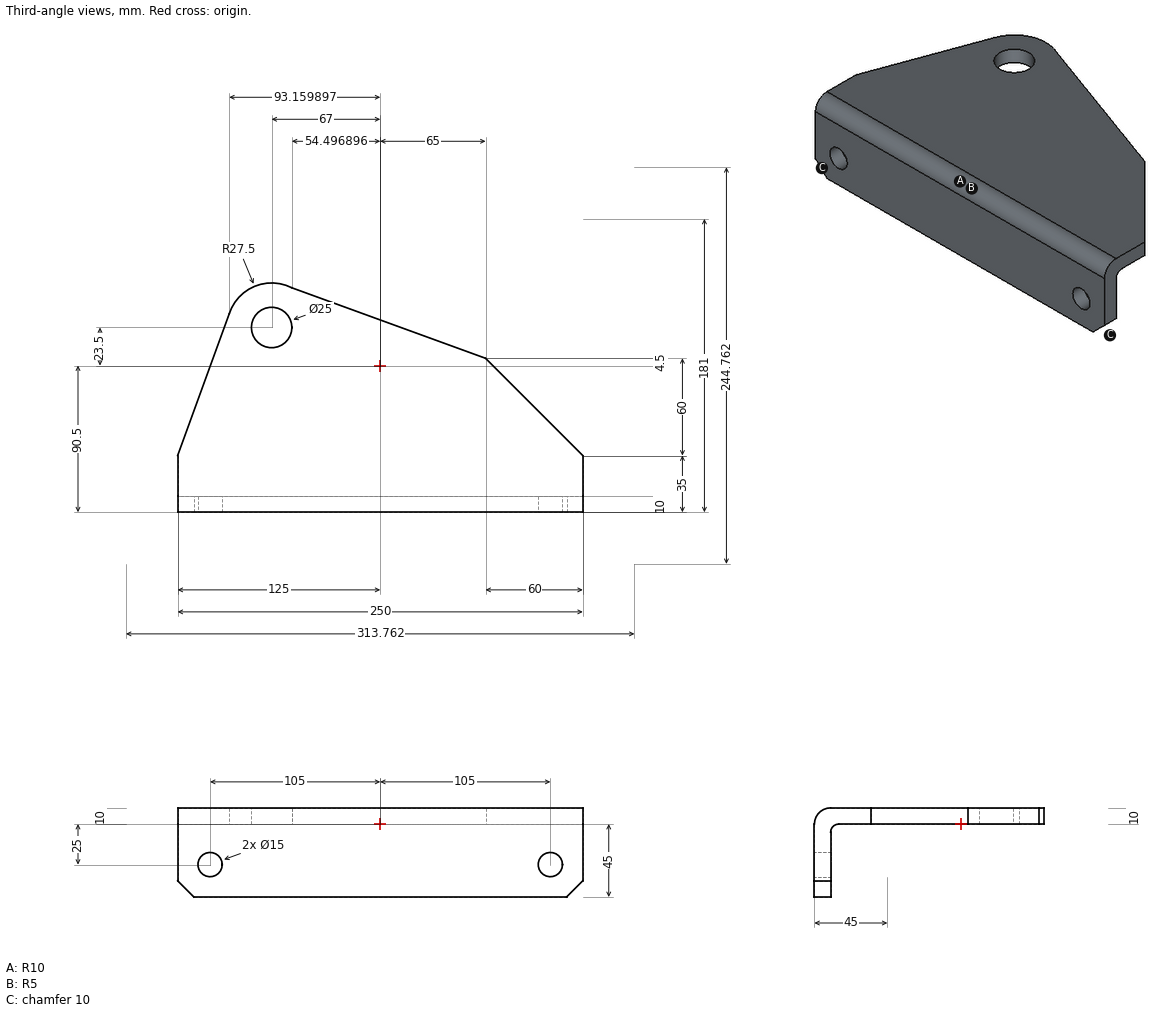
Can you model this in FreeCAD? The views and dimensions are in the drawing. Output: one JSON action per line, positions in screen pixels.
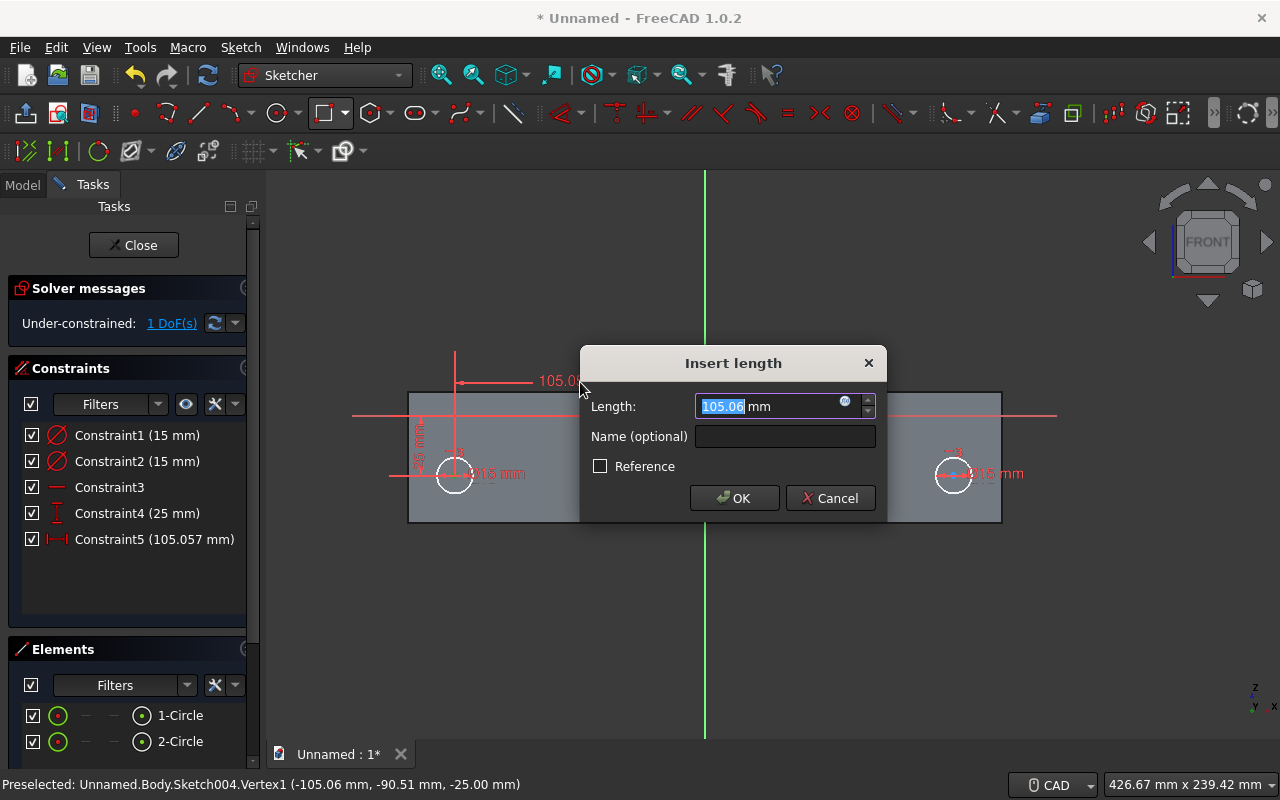
{"action": "type", "text": "105"}
{"action": "key", "text": "Return"}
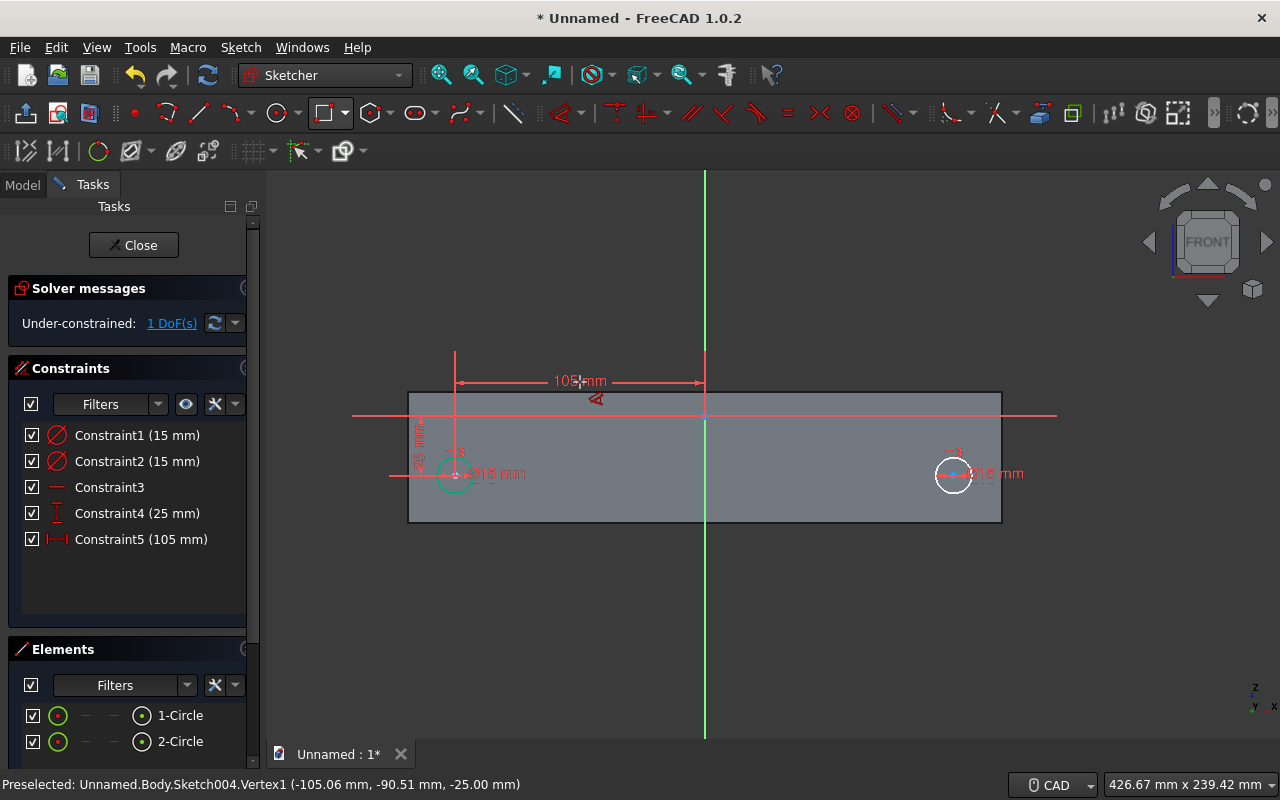
{"action": "left_click", "coordinate": [954, 476]}
{"action": "left_click", "coordinate": [829, 382]}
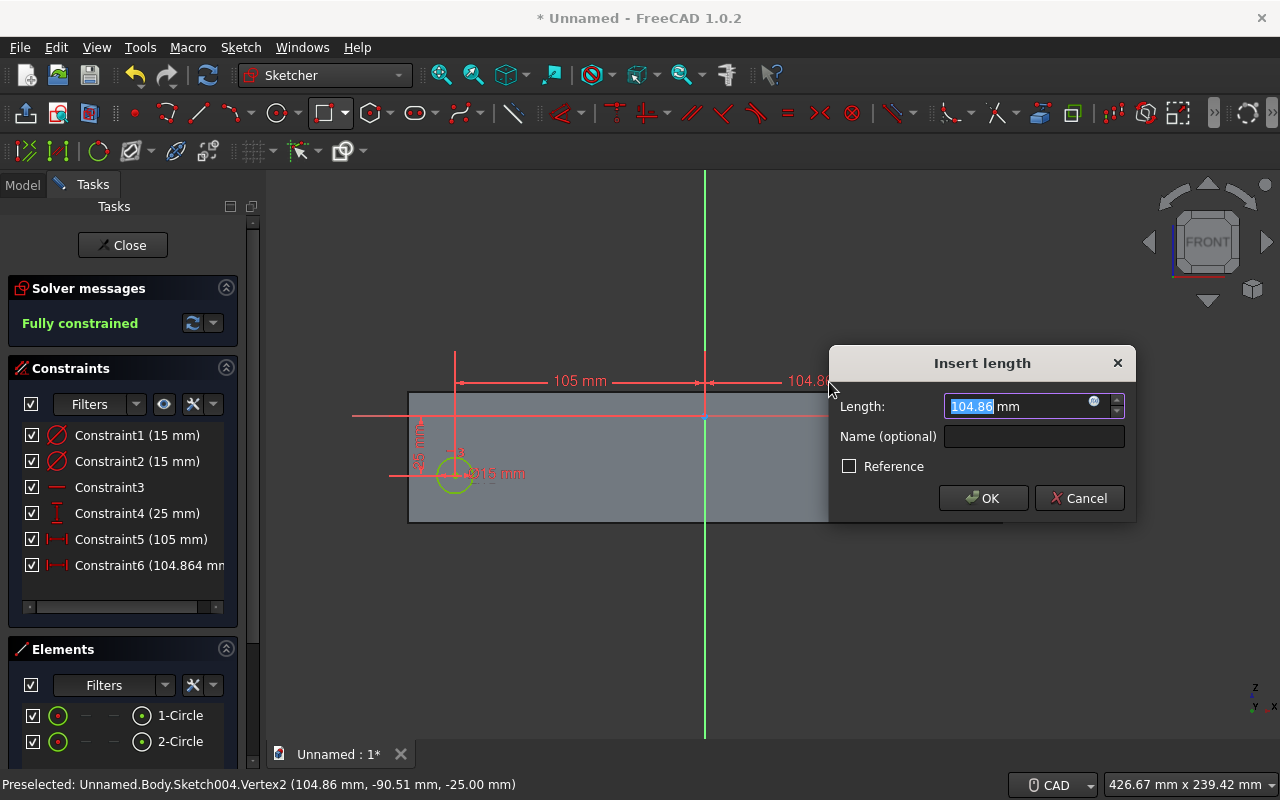
{"action": "type", "text": "105"}
{"action": "key", "text": "Return"}
{"action": "key", "text": "Escape"}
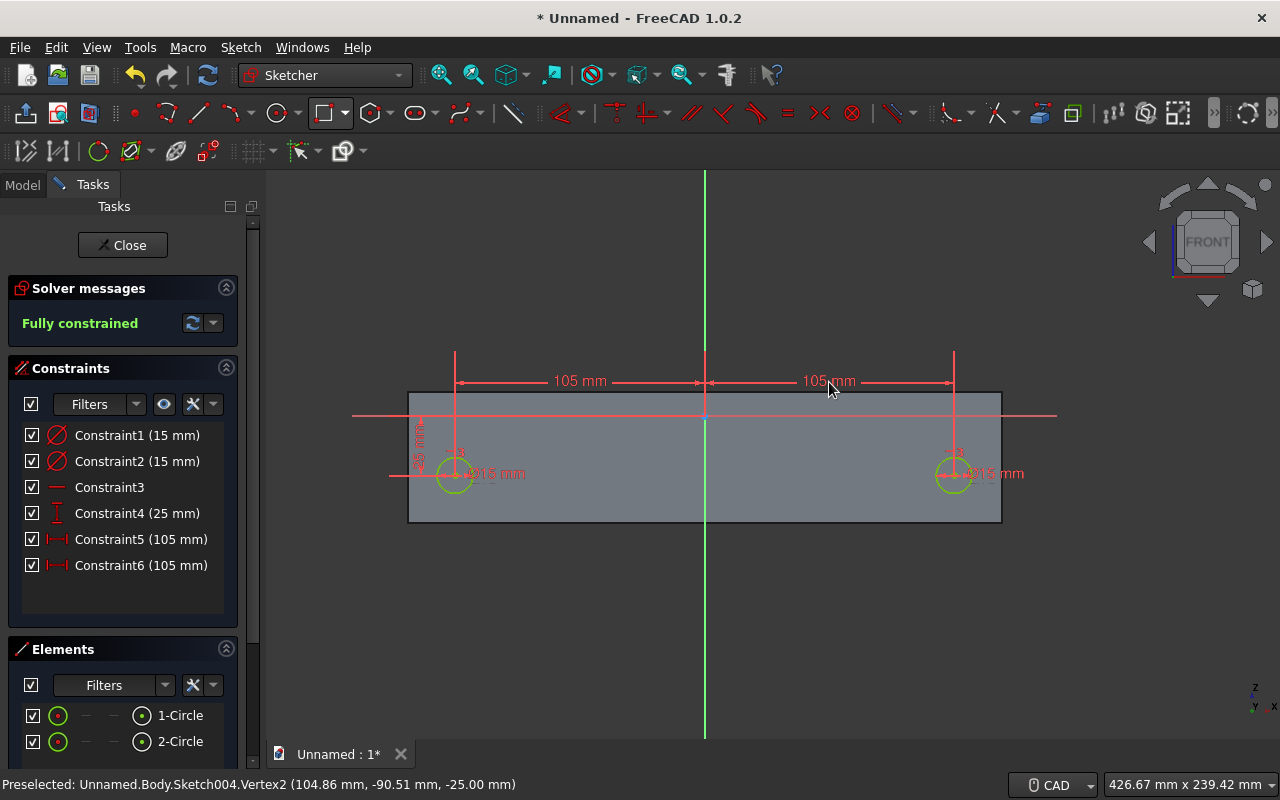
{"action": "left_click", "coordinate": [123, 245]}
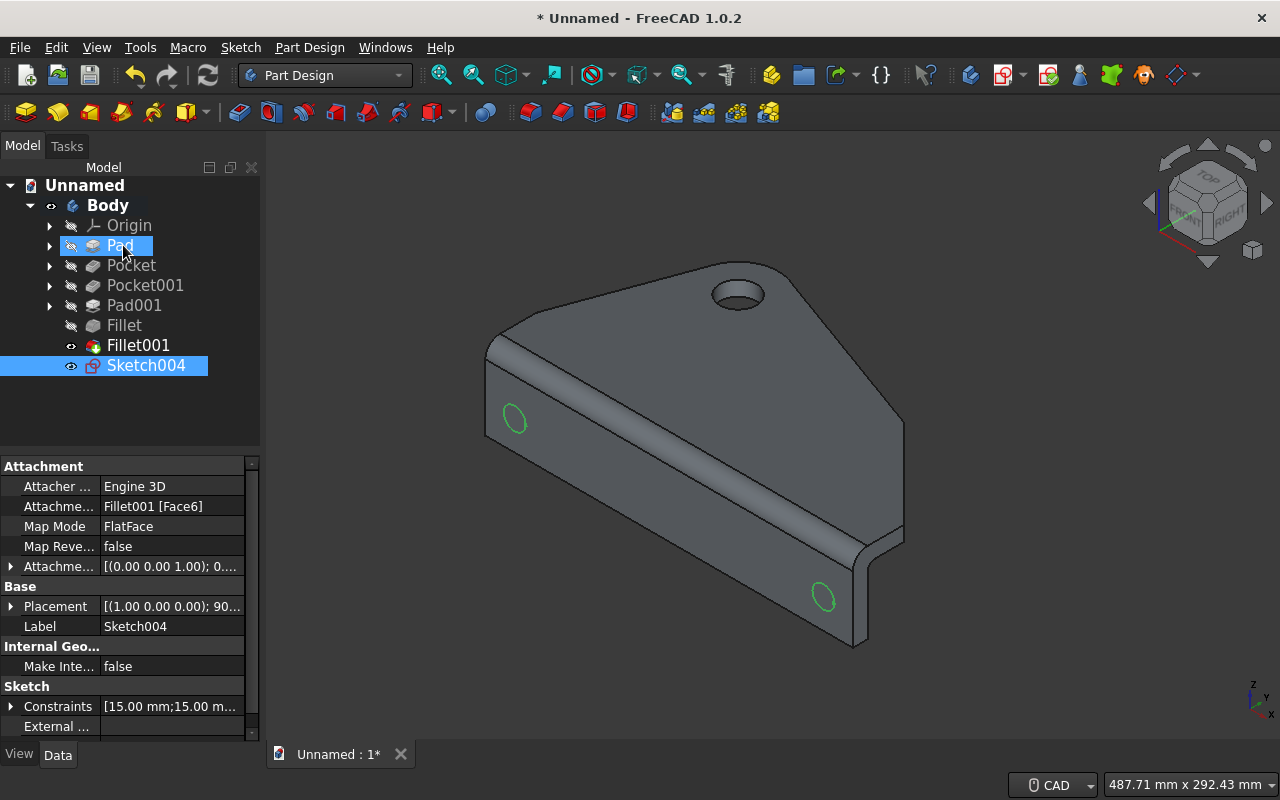
{"action": "left_click", "coordinate": [240, 112]}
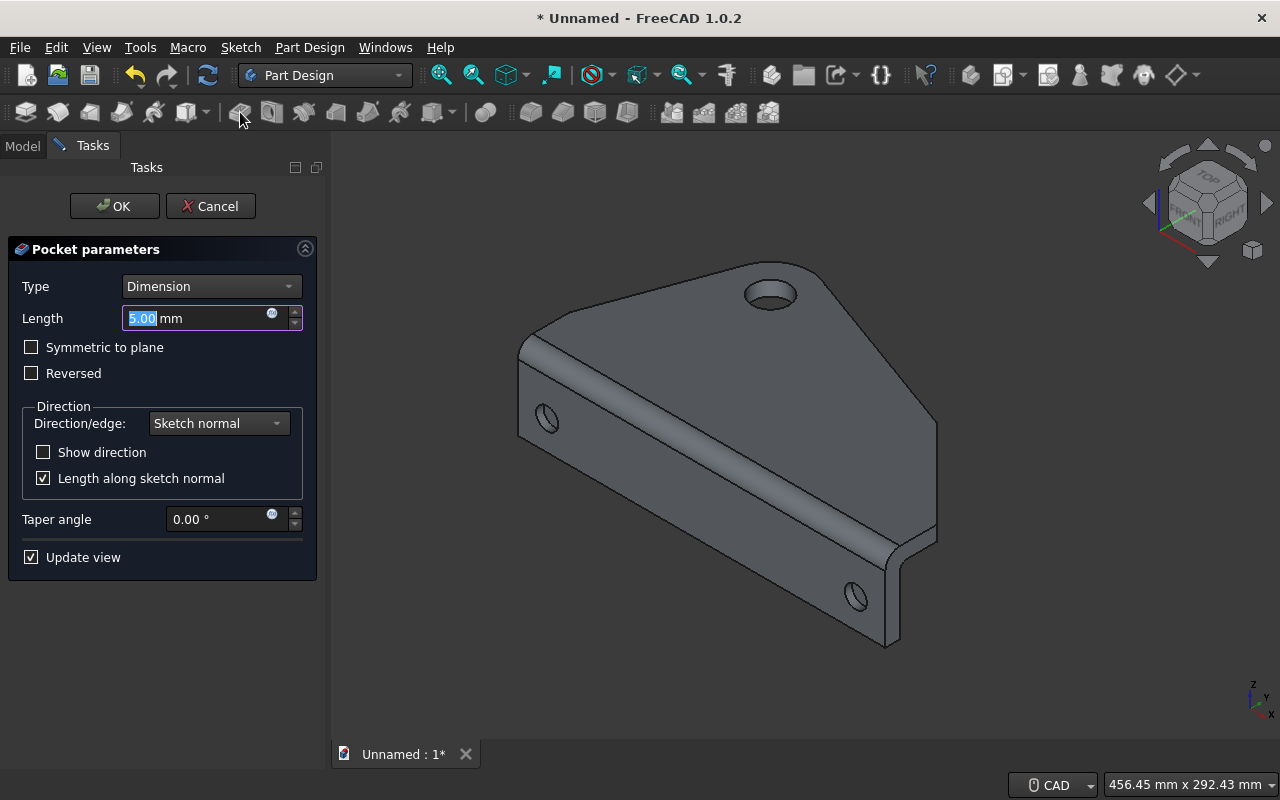
{"action": "type", "text": "45"}
{"action": "key", "text": "Tab"}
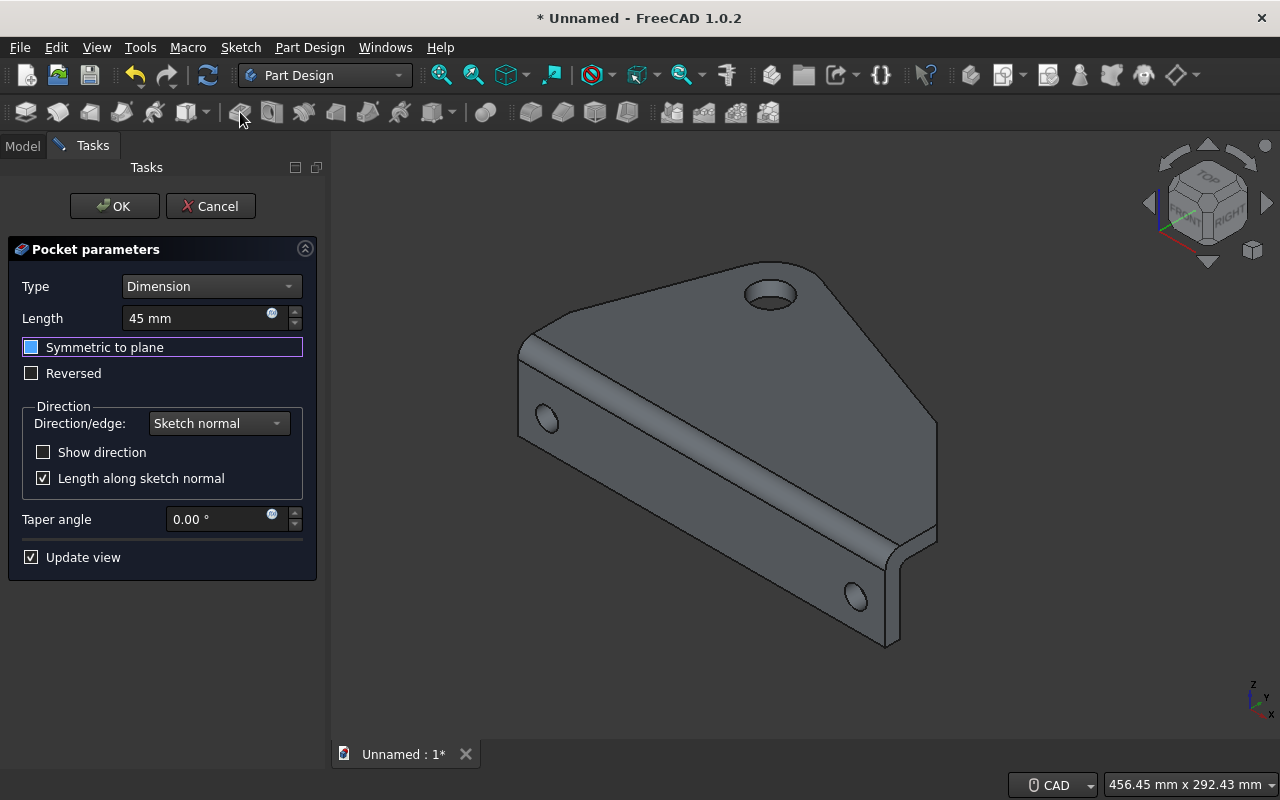
{"action": "left_click", "coordinate": [115, 206]}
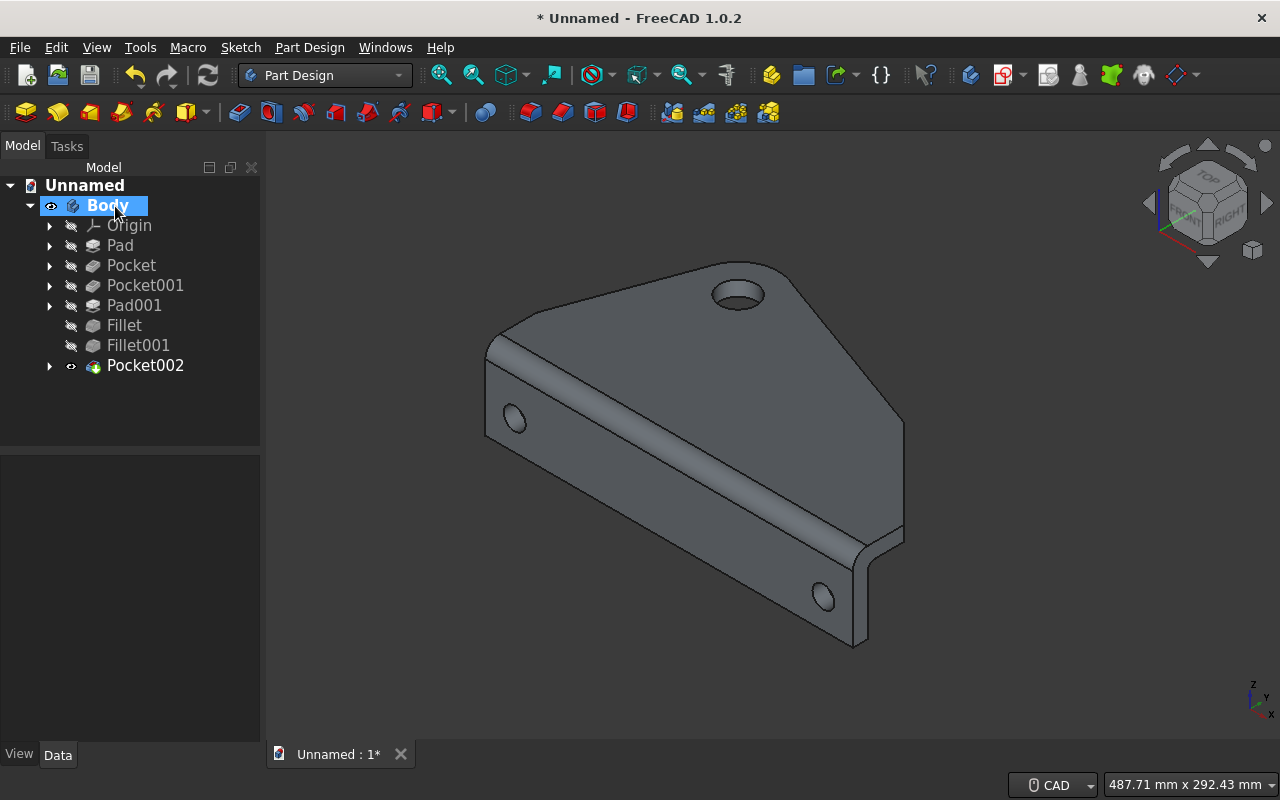
{"action": "scroll", "coordinate": [860, 643], "scroll_direction": "up", "scroll_amount": 4}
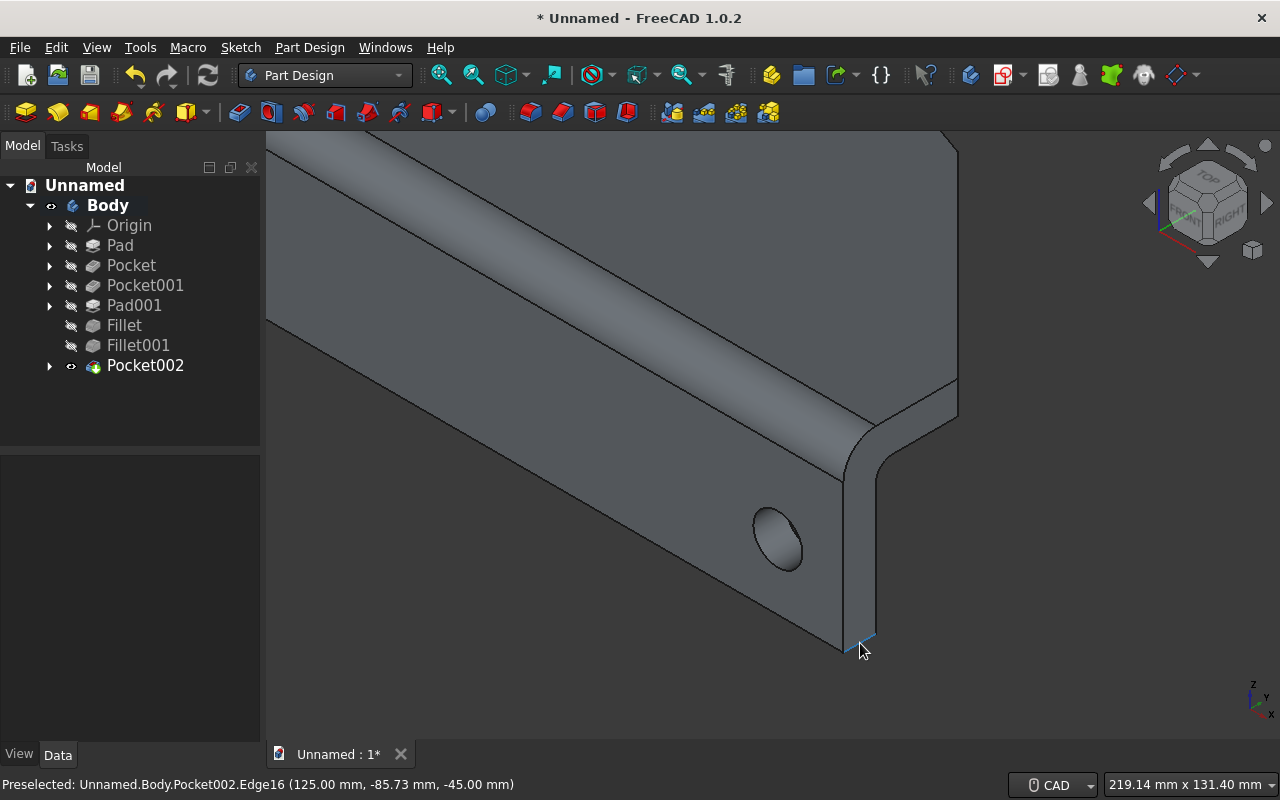
{"action": "key", "text": "v f"}